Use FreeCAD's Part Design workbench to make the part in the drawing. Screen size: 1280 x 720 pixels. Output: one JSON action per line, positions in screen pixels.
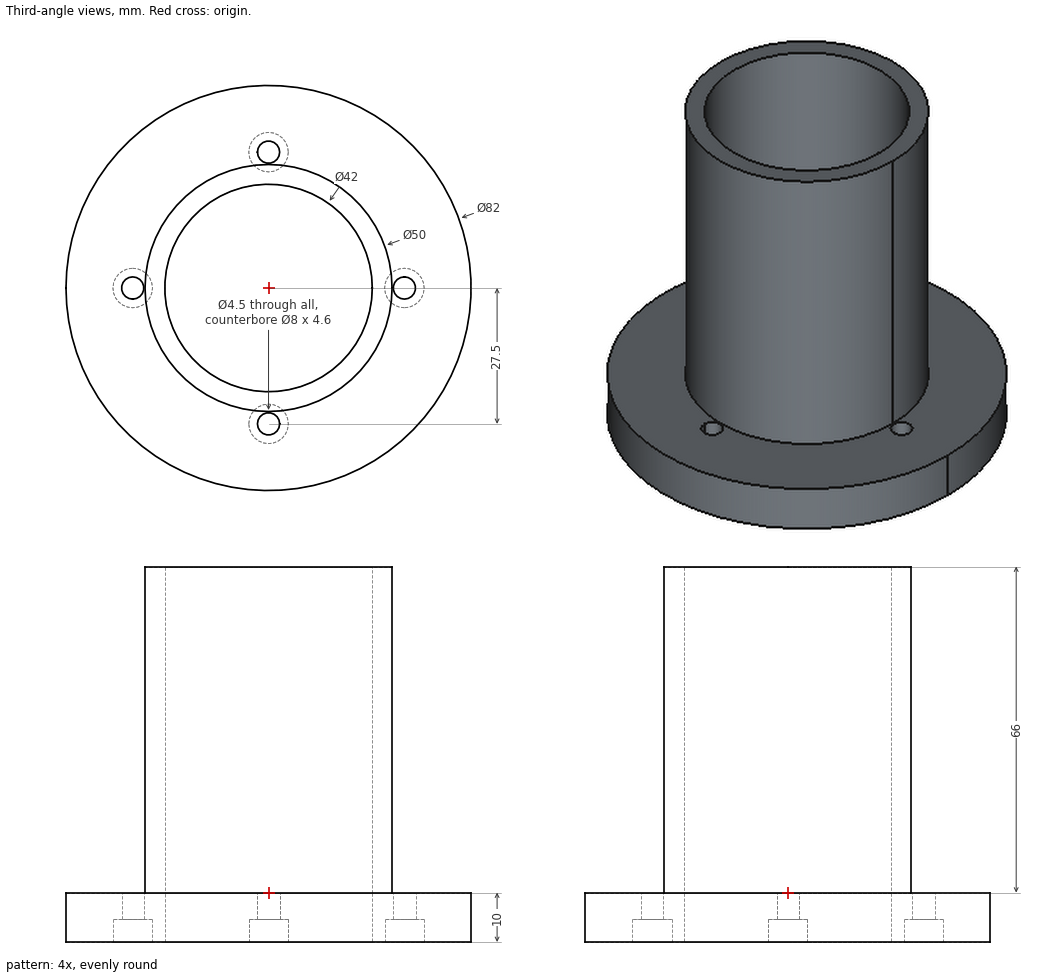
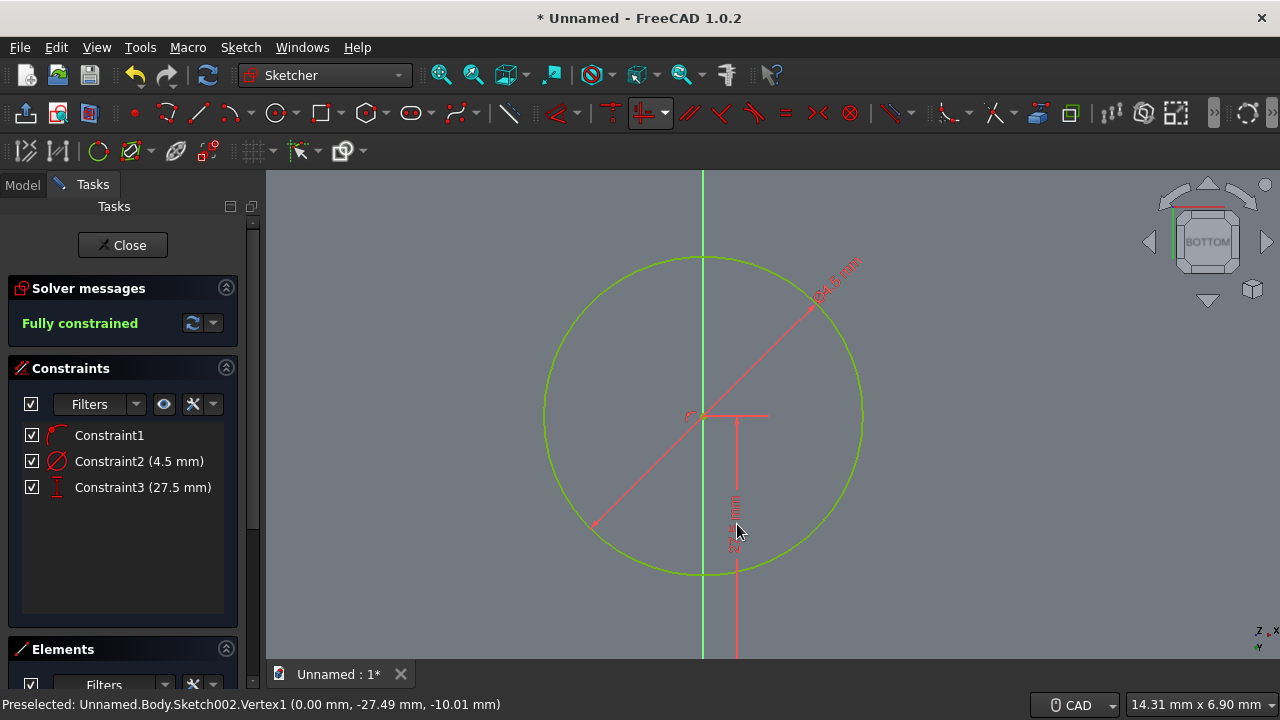
{"action": "left_click", "coordinate": [123, 245]}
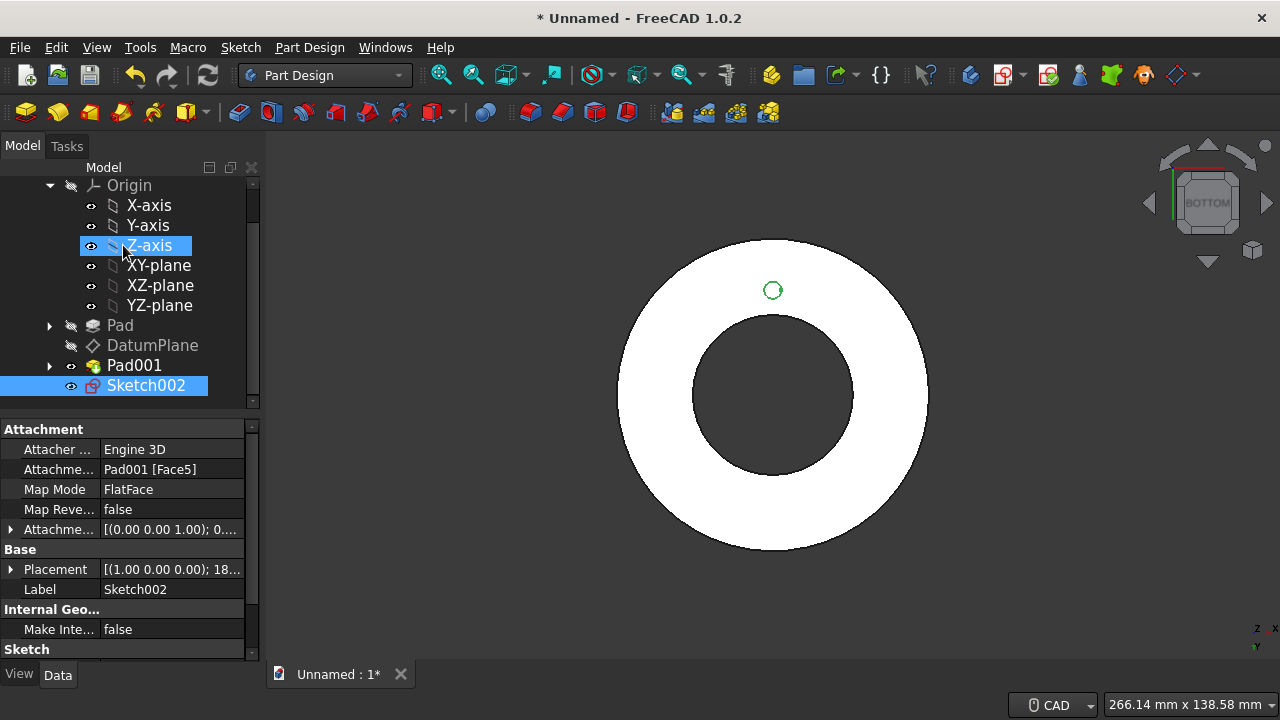
{"action": "left_click", "coordinate": [272, 112]}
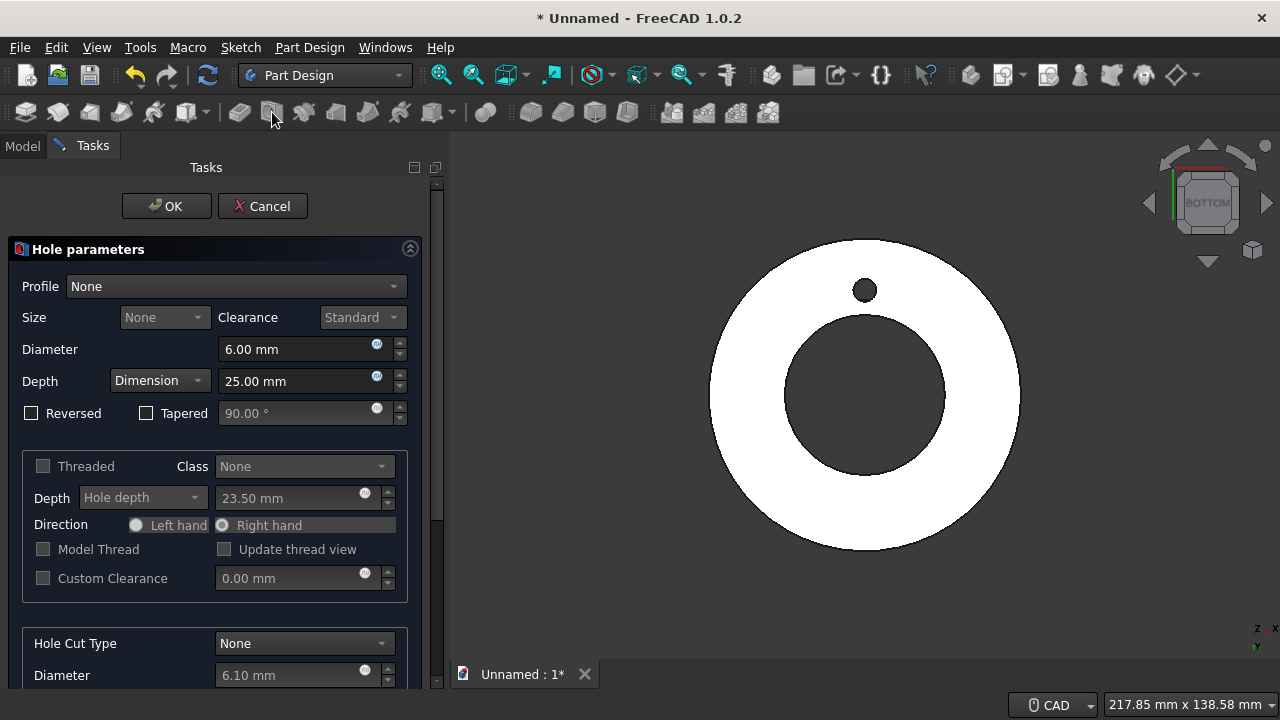
{"action": "triple_click", "coordinate": [305, 349]}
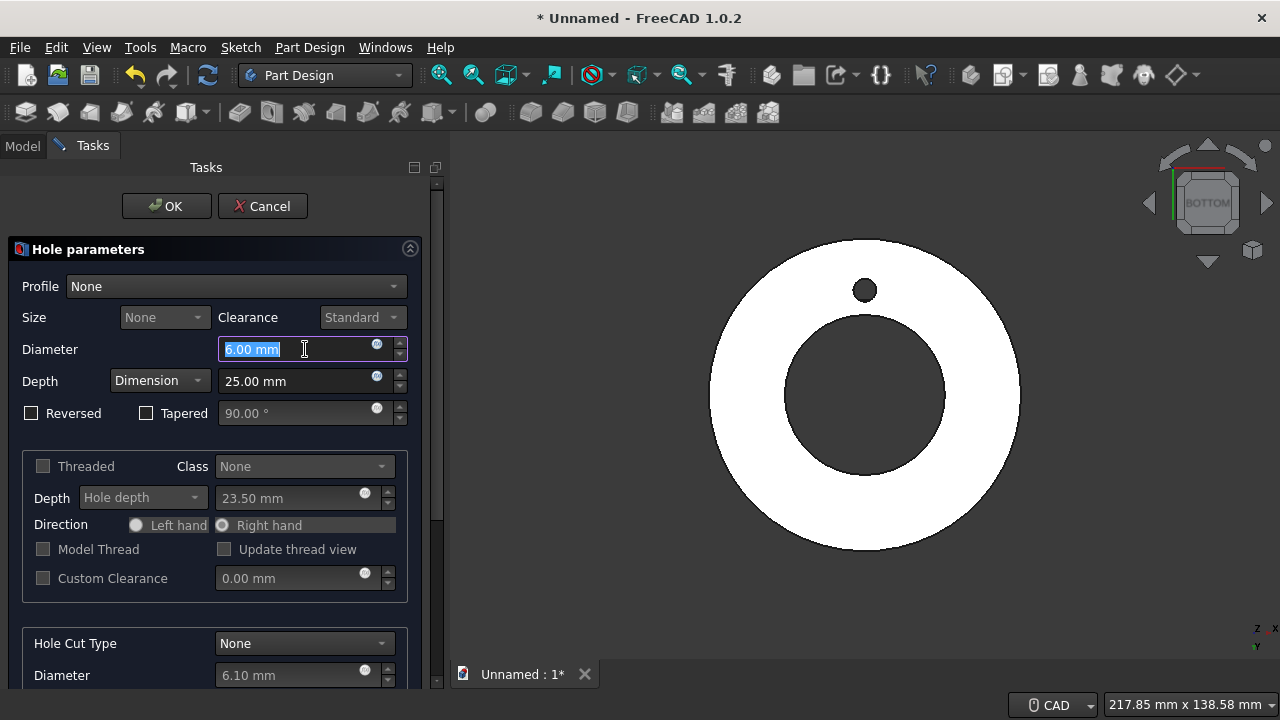
{"action": "type", "text": "4.5"}
{"action": "key", "text": "Tab"}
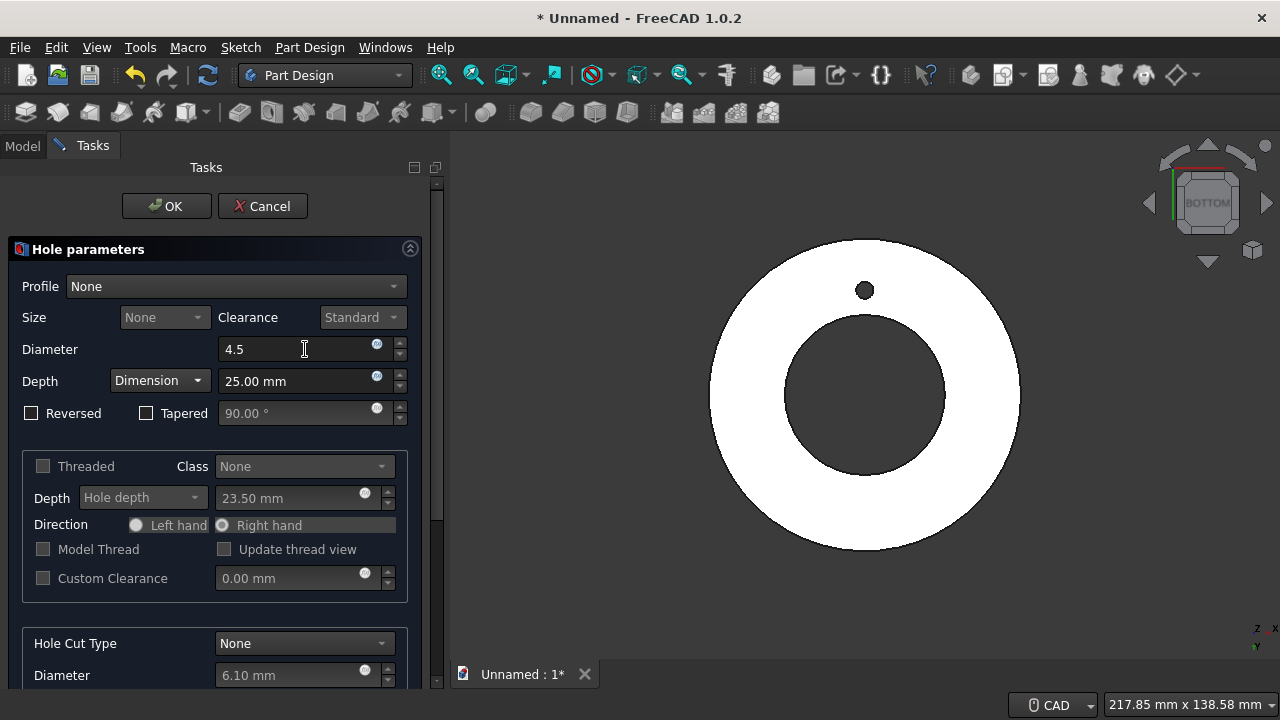
{"action": "left_click", "coordinate": [161, 380]}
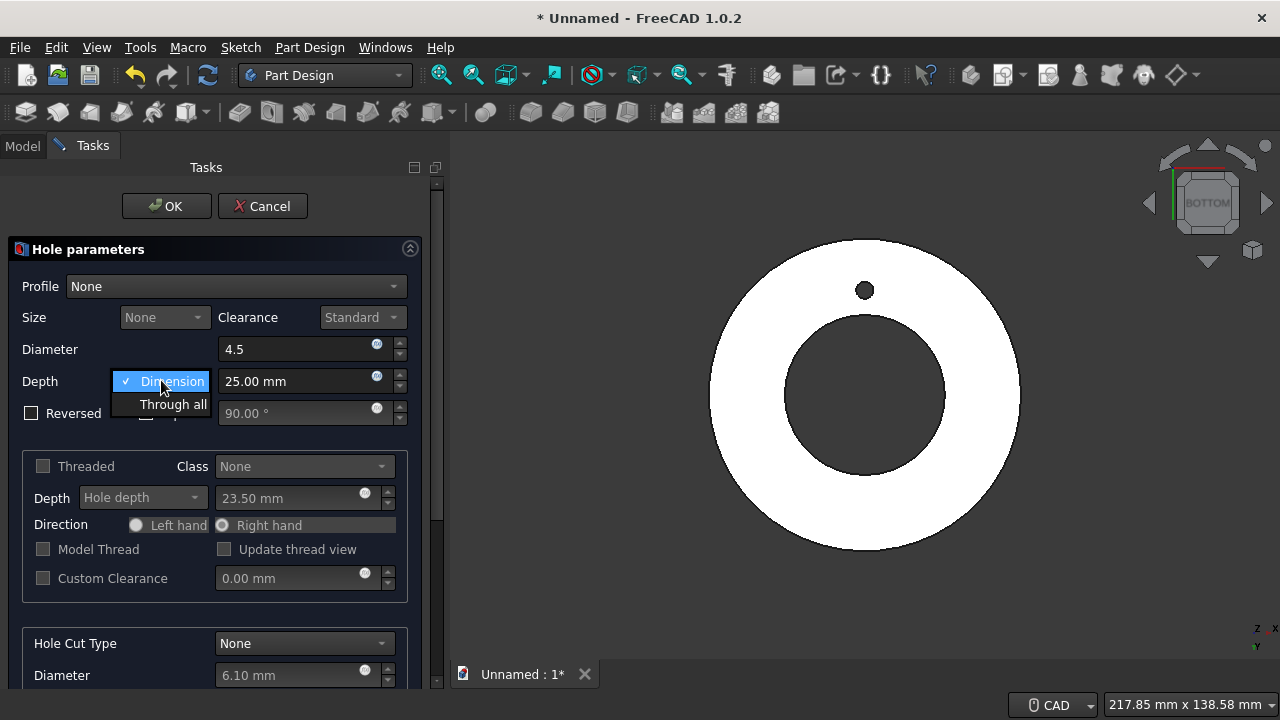
{"action": "left_click", "coordinate": [160, 404]}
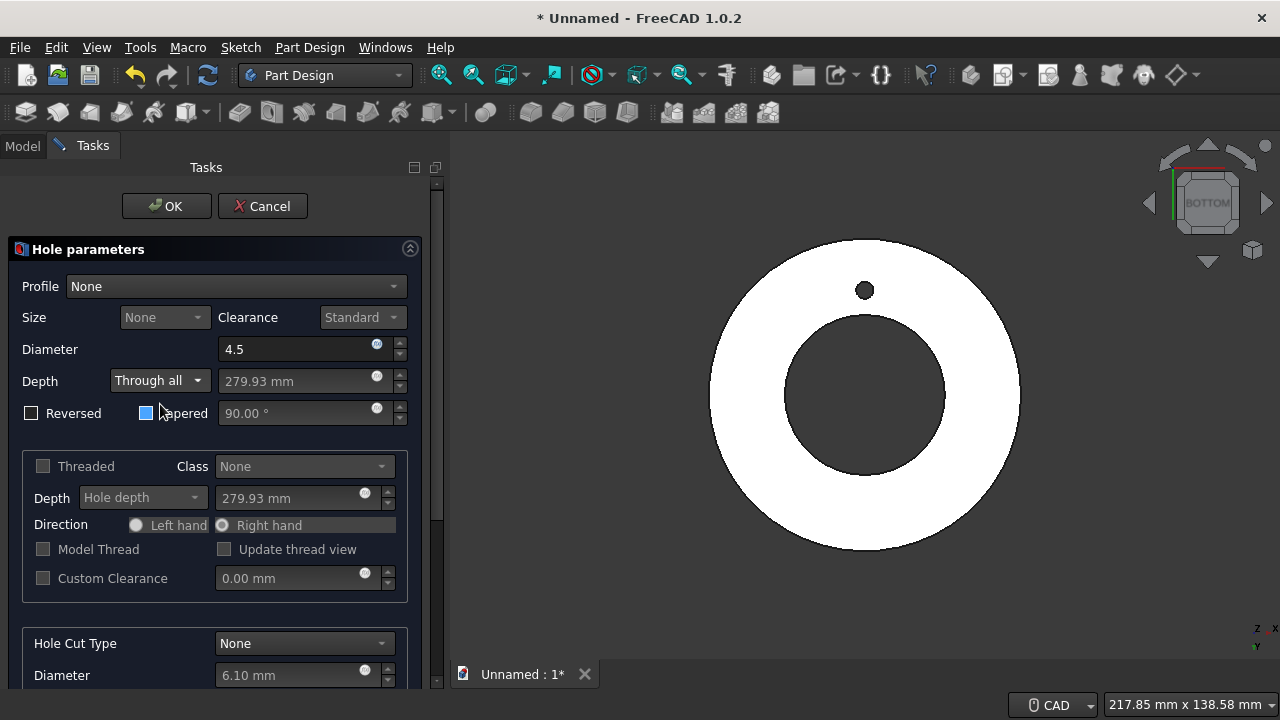
{"action": "left_click", "coordinate": [306, 644]}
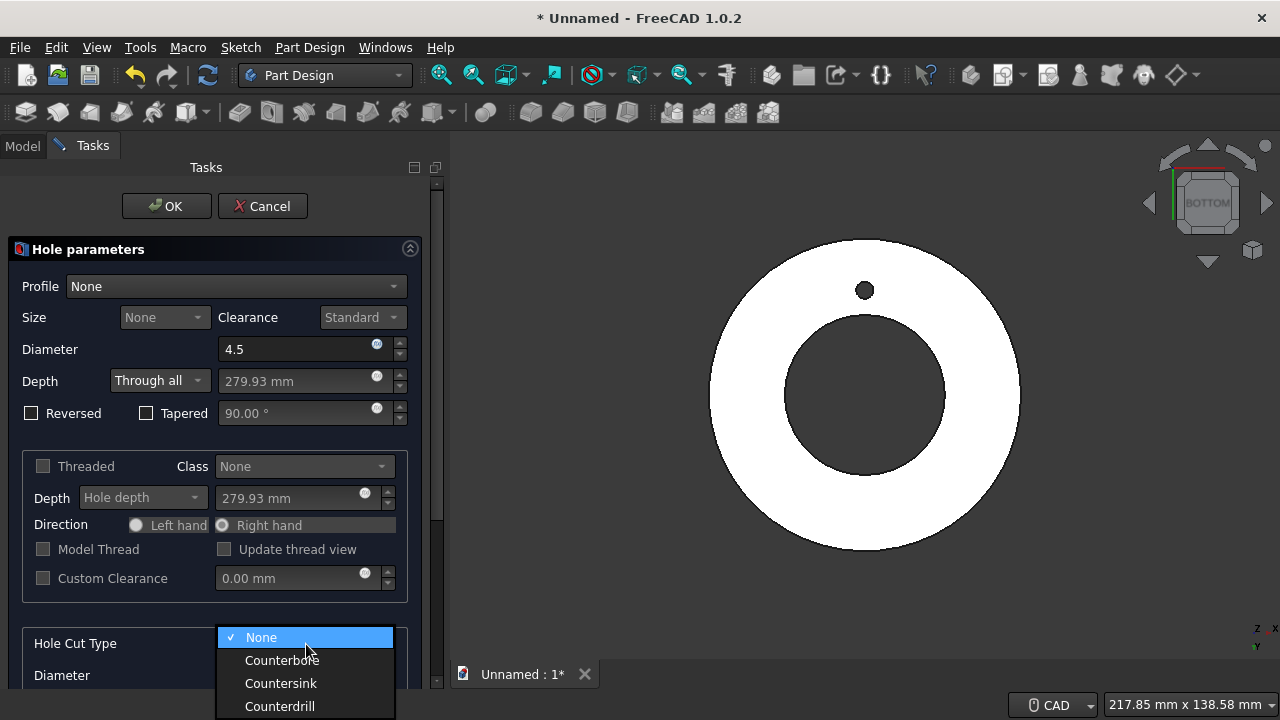
{"action": "left_click", "coordinate": [304, 660]}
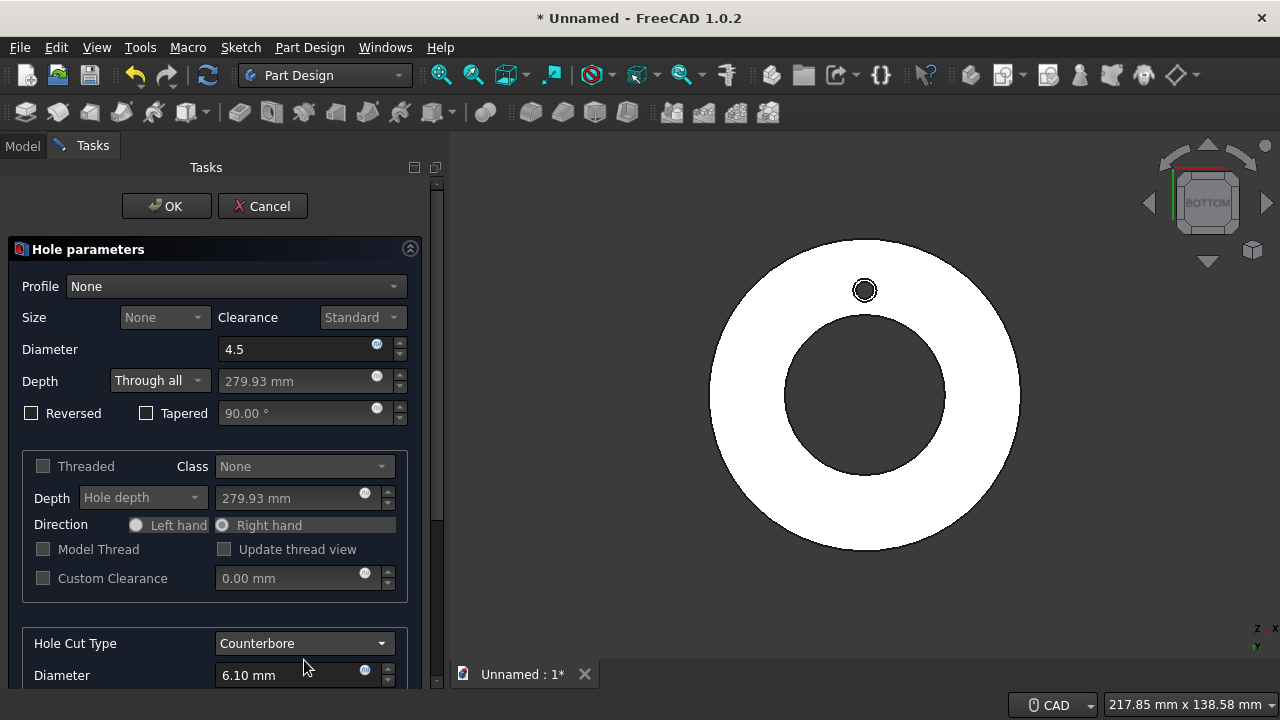
{"action": "triple_click", "coordinate": [298, 675]}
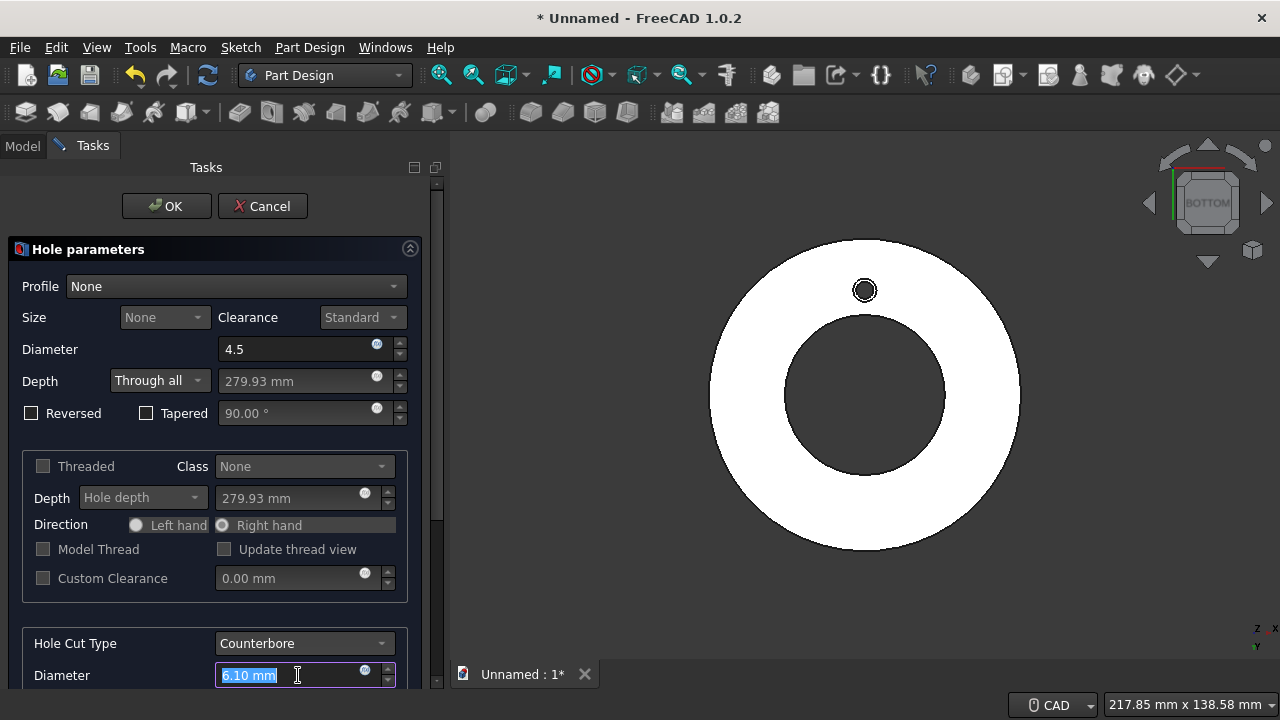
{"action": "type", "text": "8"}
{"action": "key", "text": "Tab"}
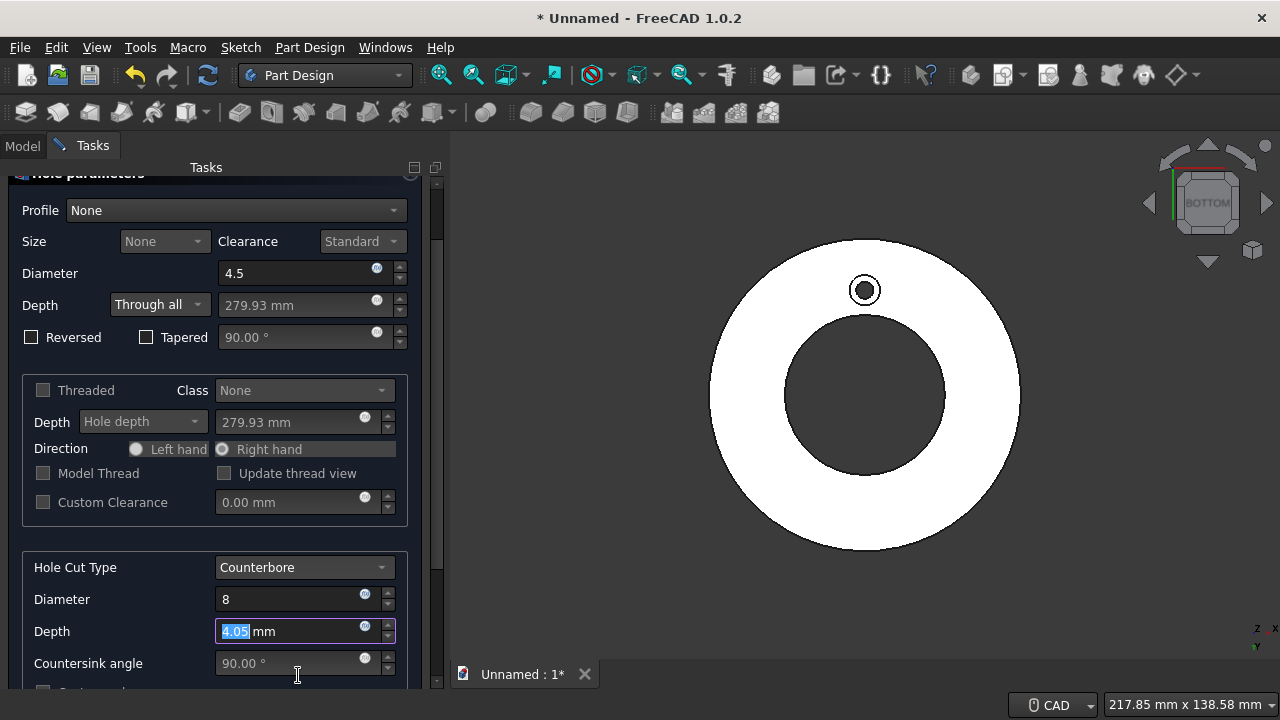
{"action": "type", "text": "4.6"}
{"action": "key", "text": "Tab"}